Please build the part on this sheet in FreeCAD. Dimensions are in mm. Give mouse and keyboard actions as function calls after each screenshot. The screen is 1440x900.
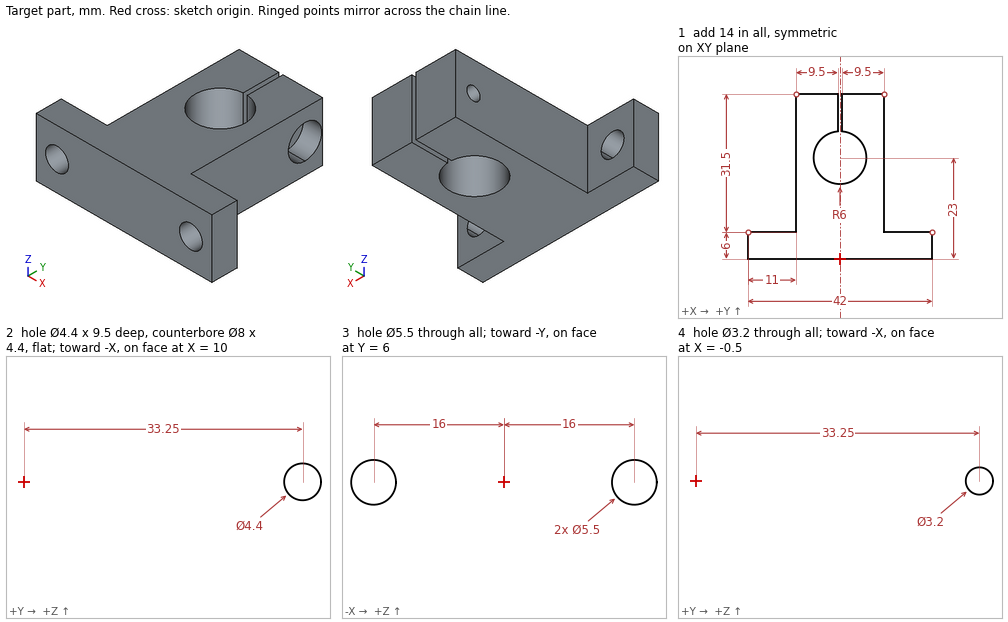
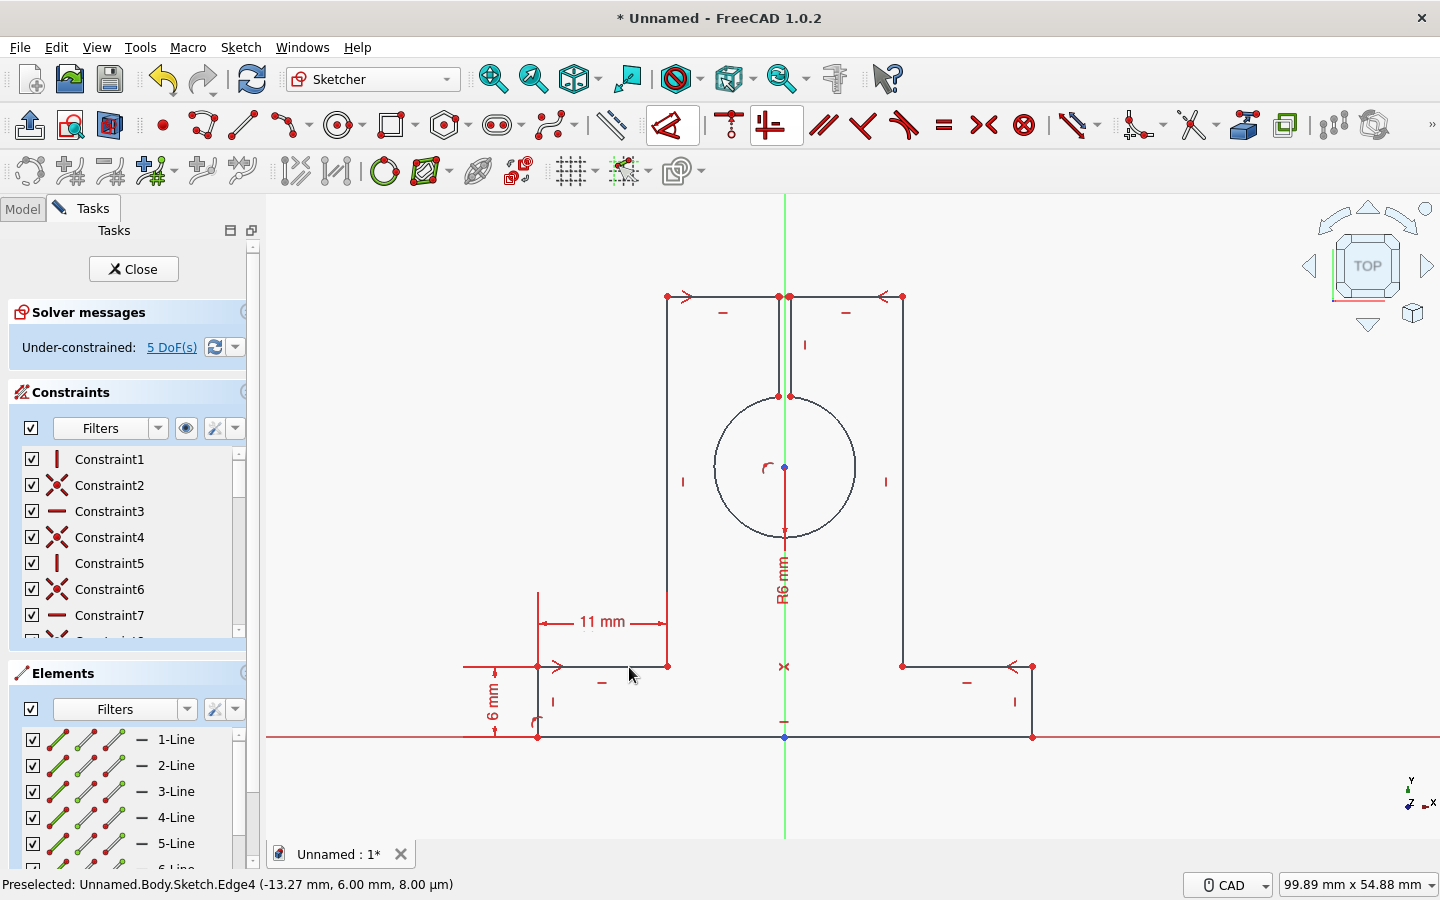
click(686, 737)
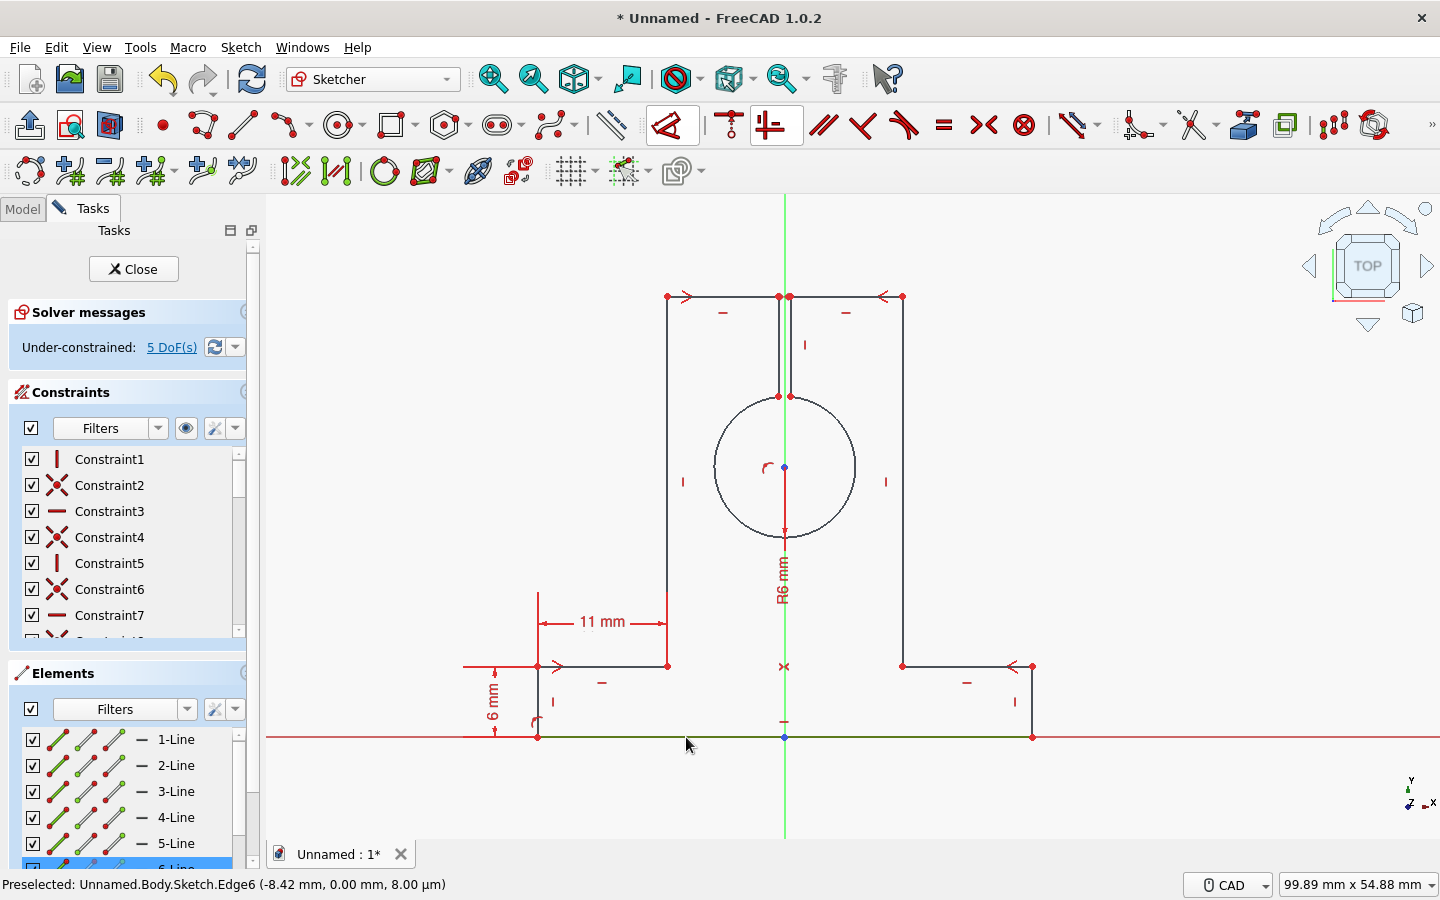
click(694, 126)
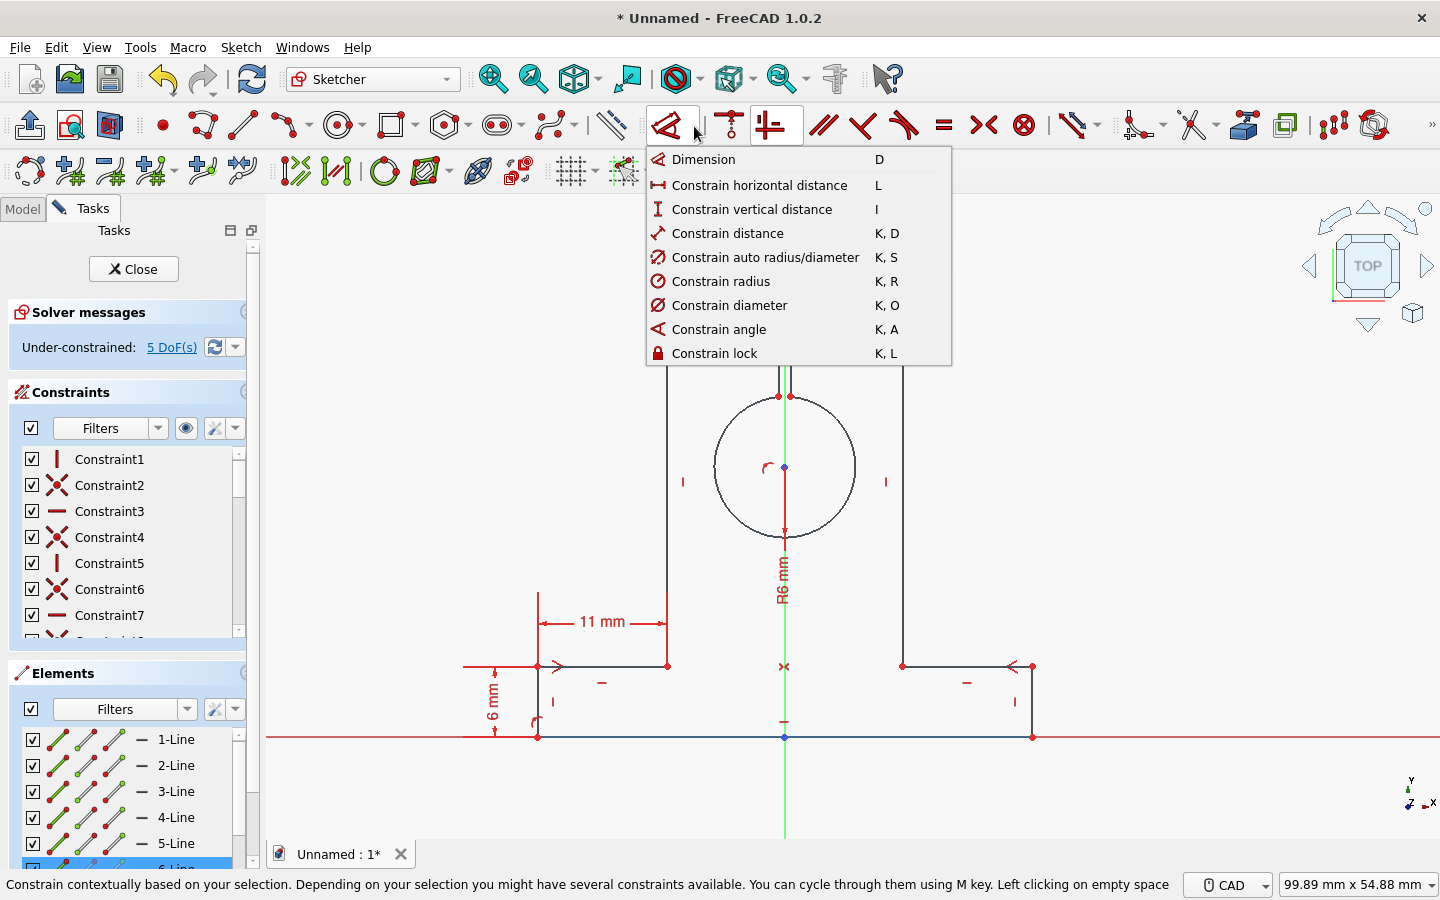
click(799, 185)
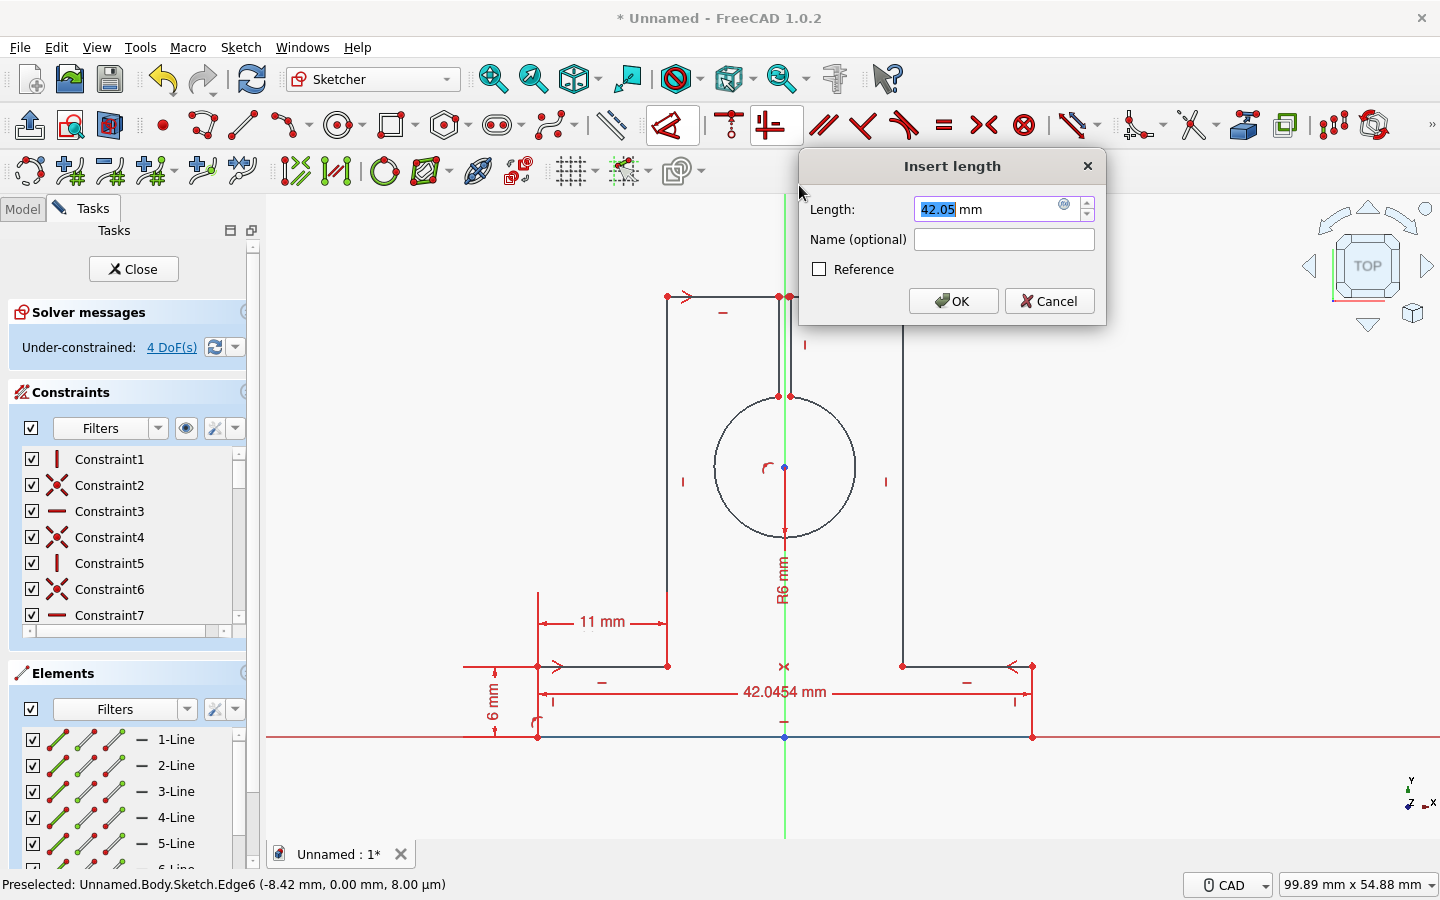
text(42)
key(Return)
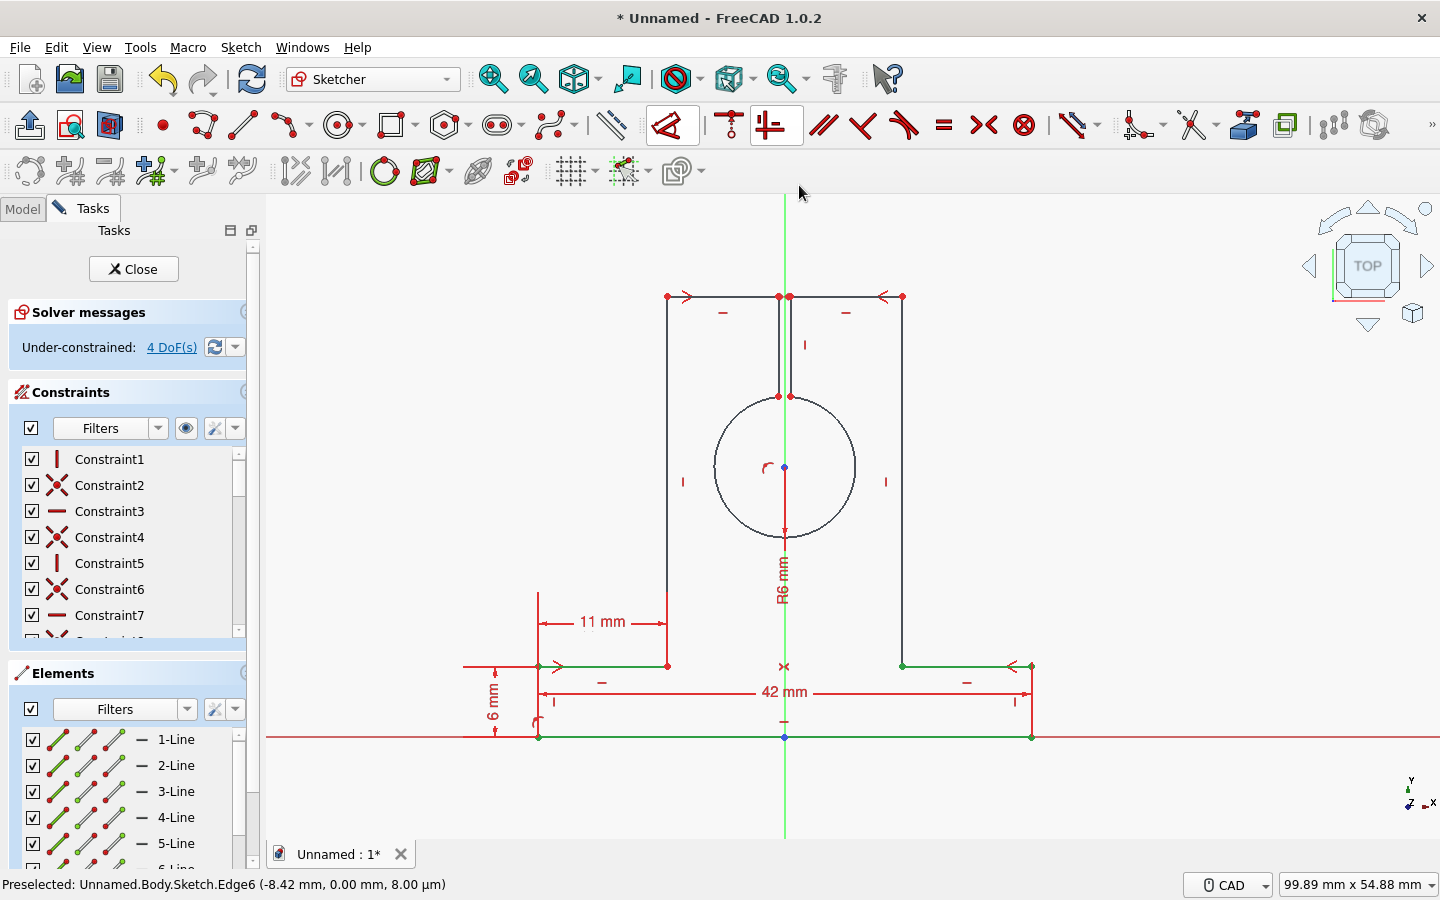
click(745, 297)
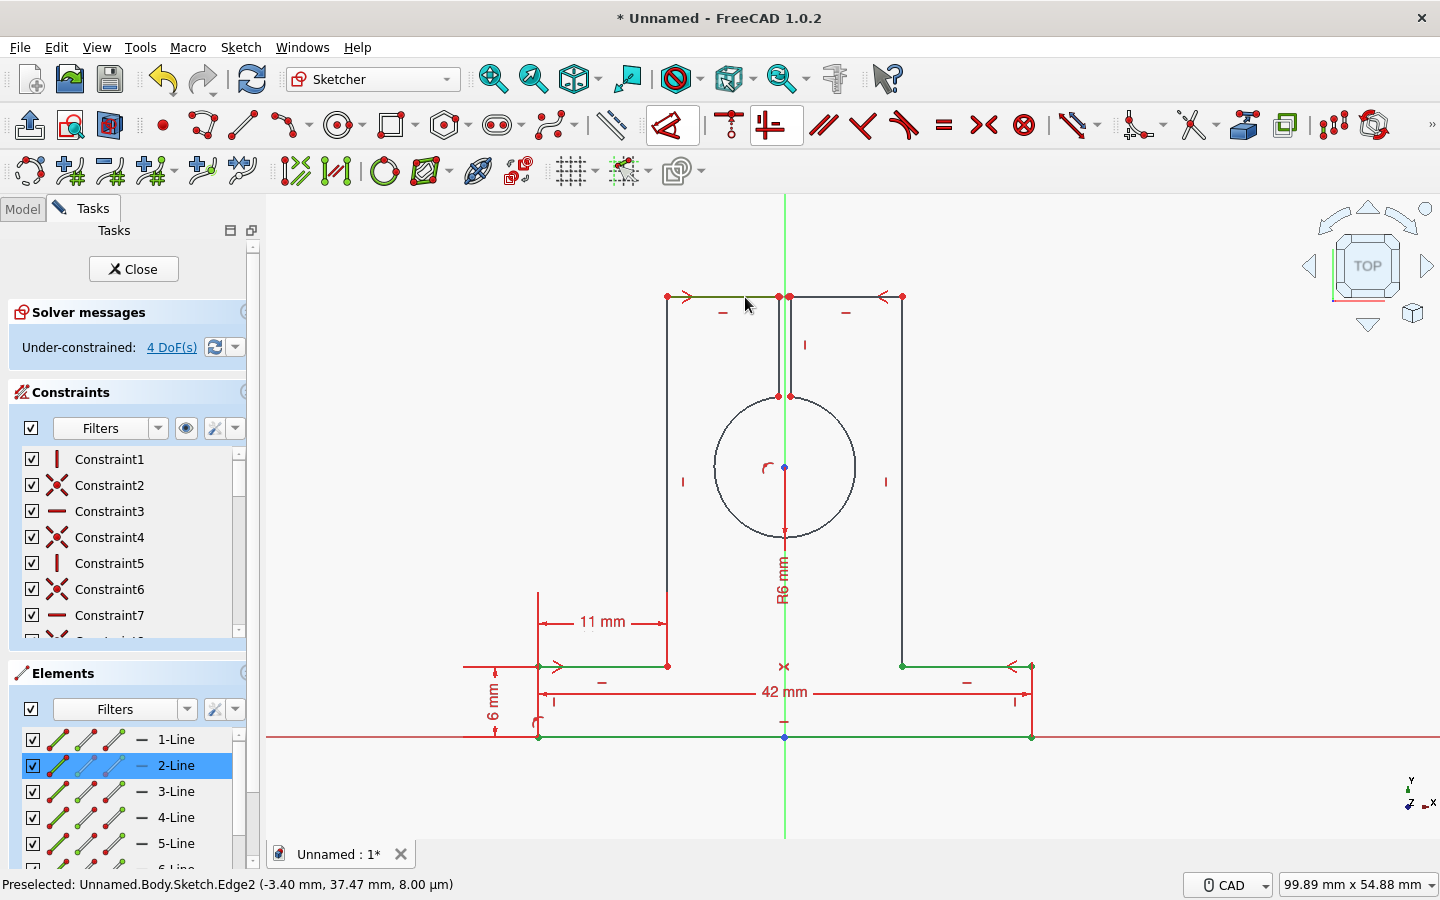
key(l)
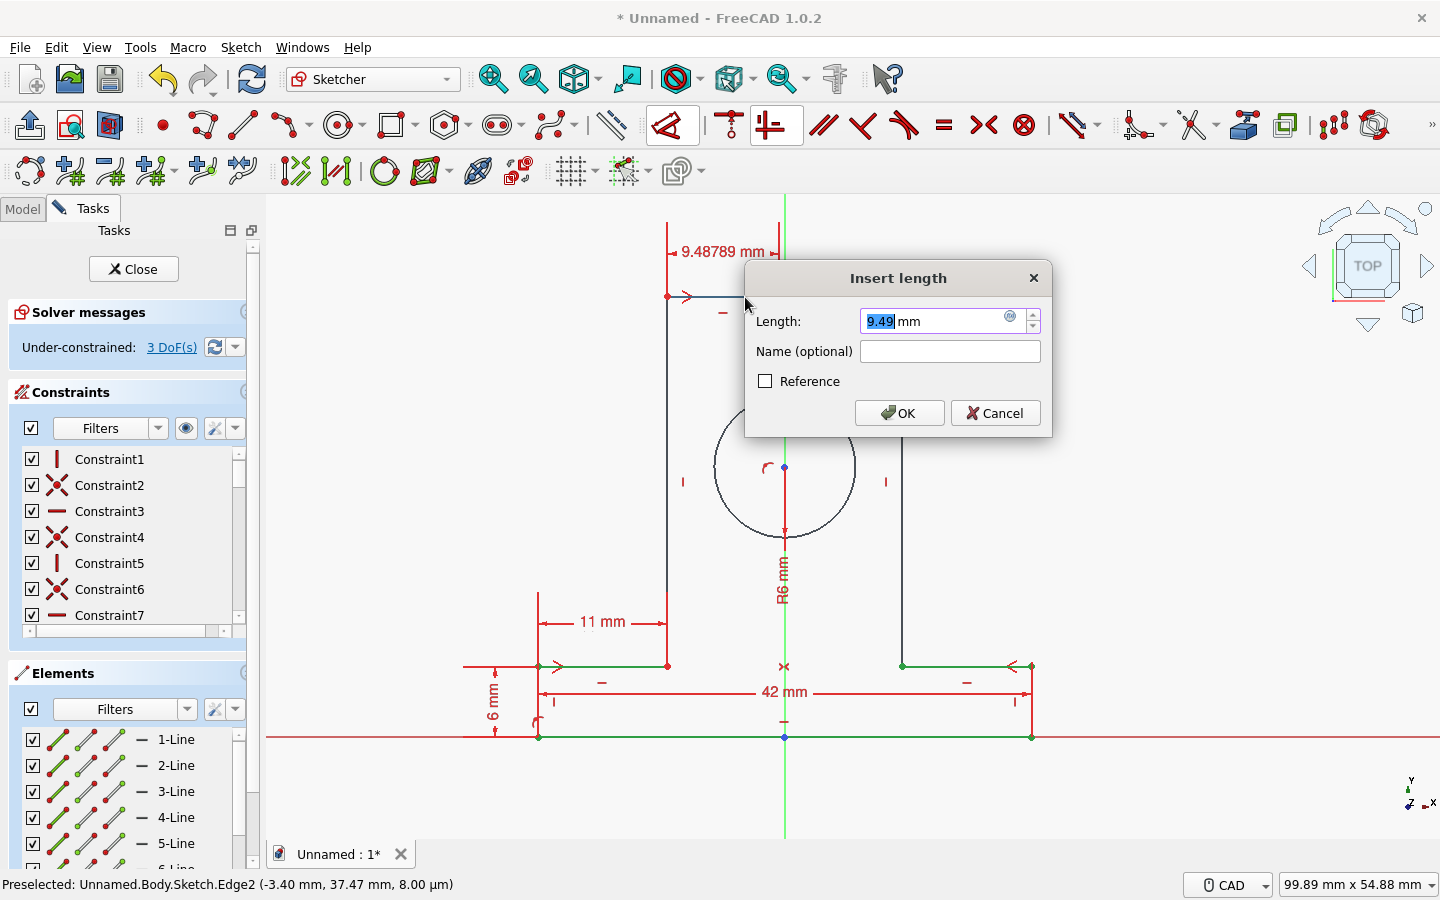
text(9.5)
key(Return)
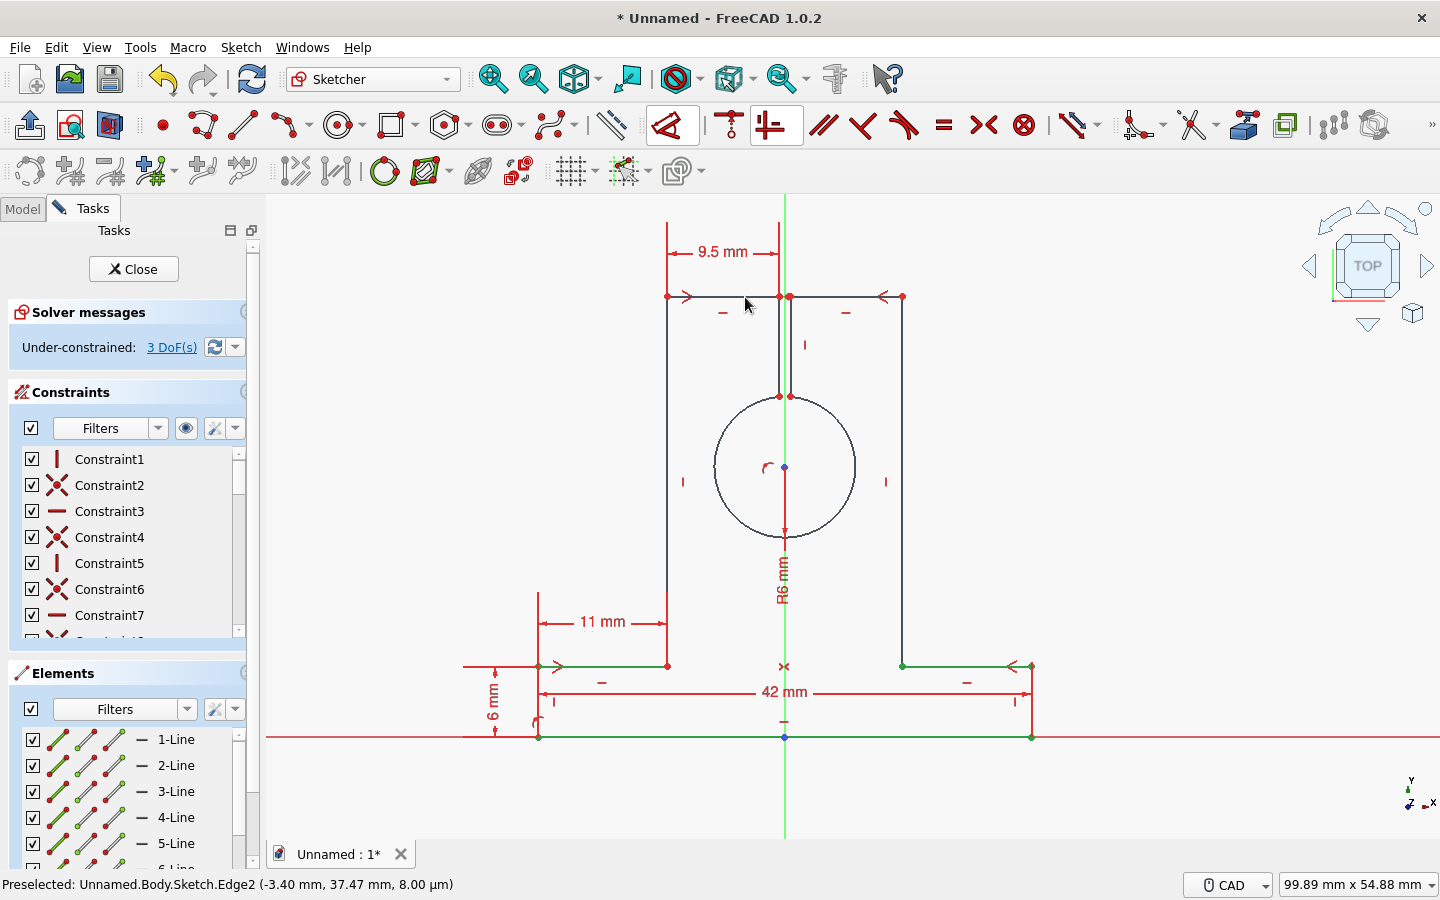
click(869, 297)